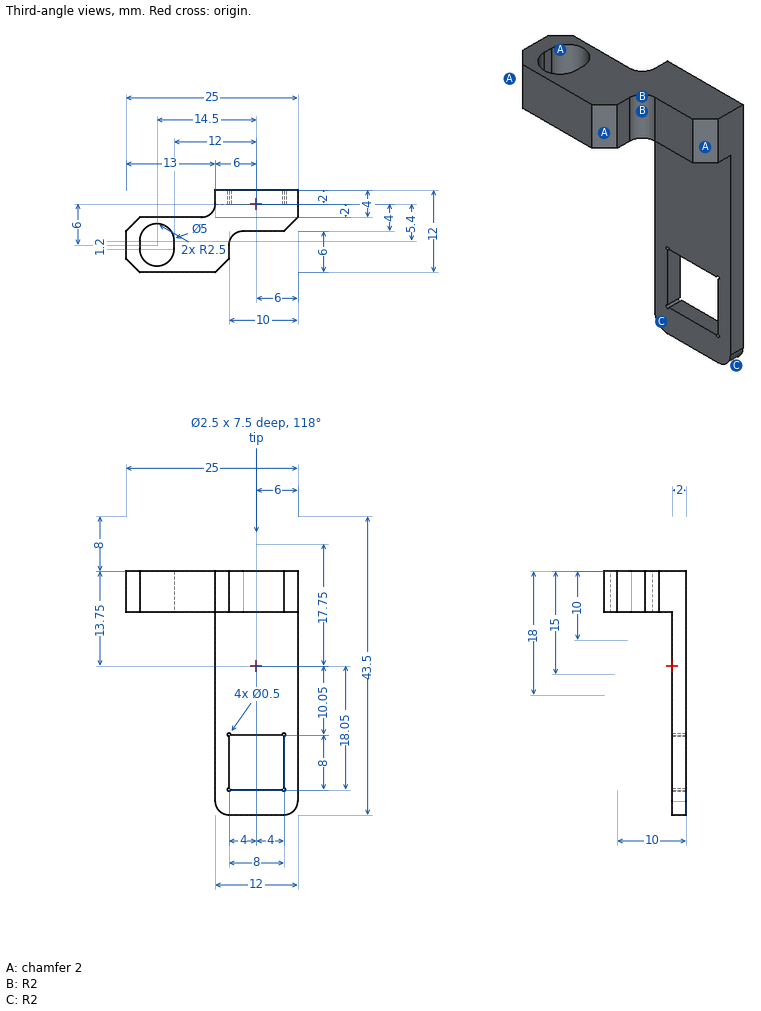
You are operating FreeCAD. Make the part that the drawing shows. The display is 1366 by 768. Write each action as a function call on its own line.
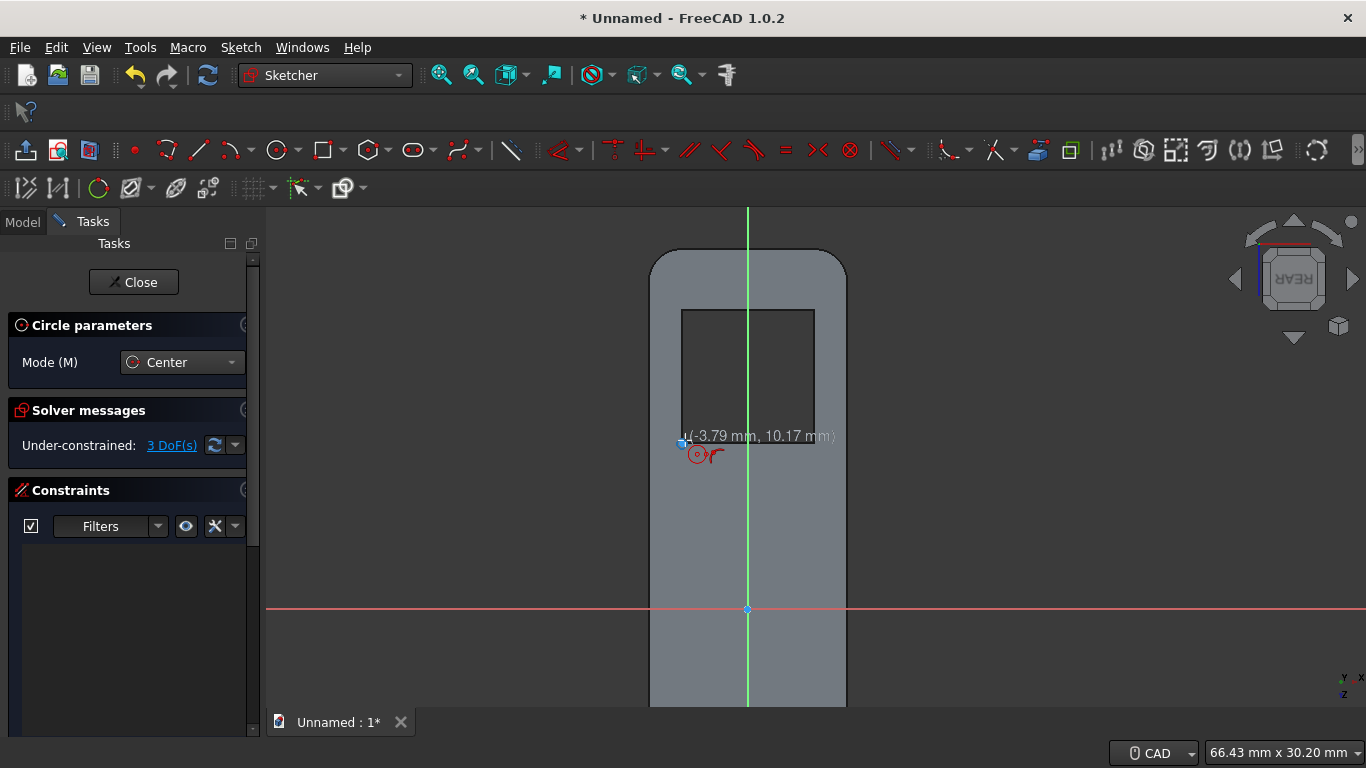
scroll(814, 443, up, 9)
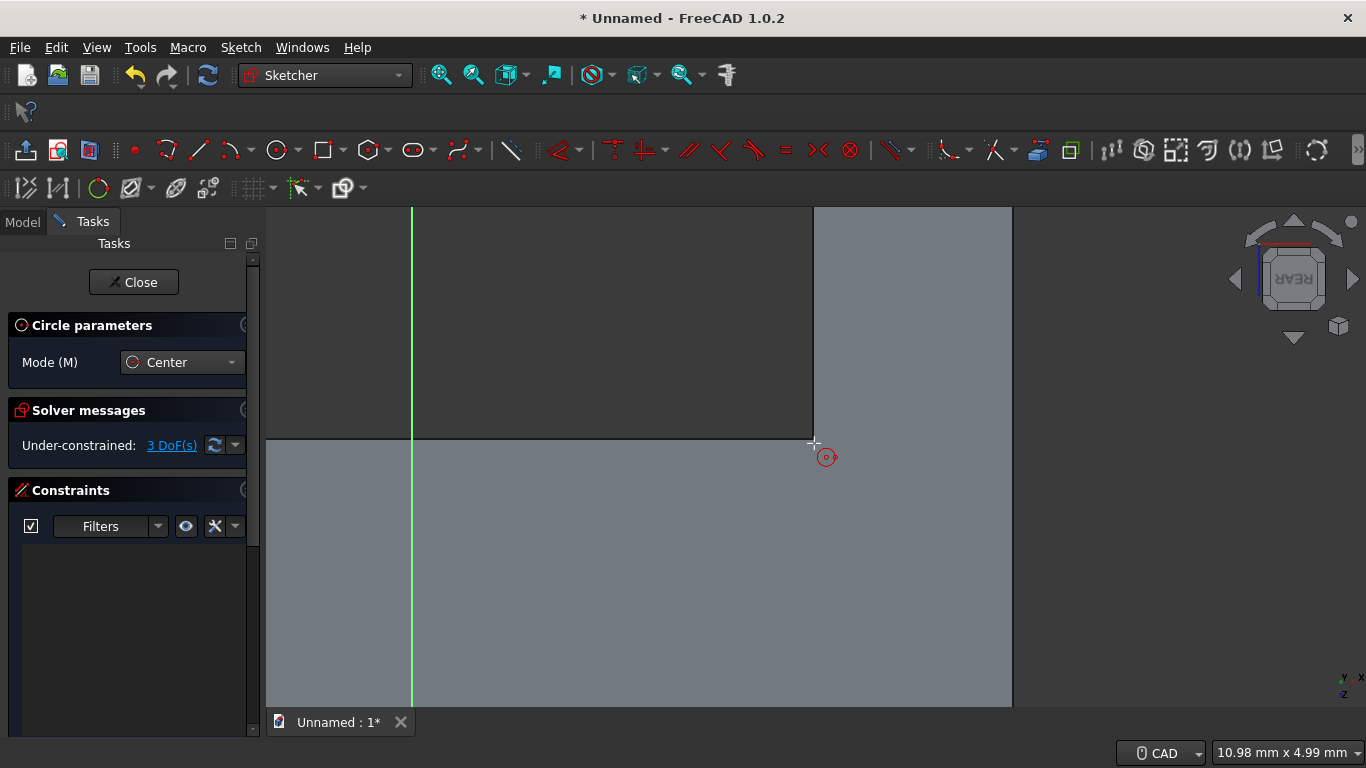
scroll(814, 443, down, 9)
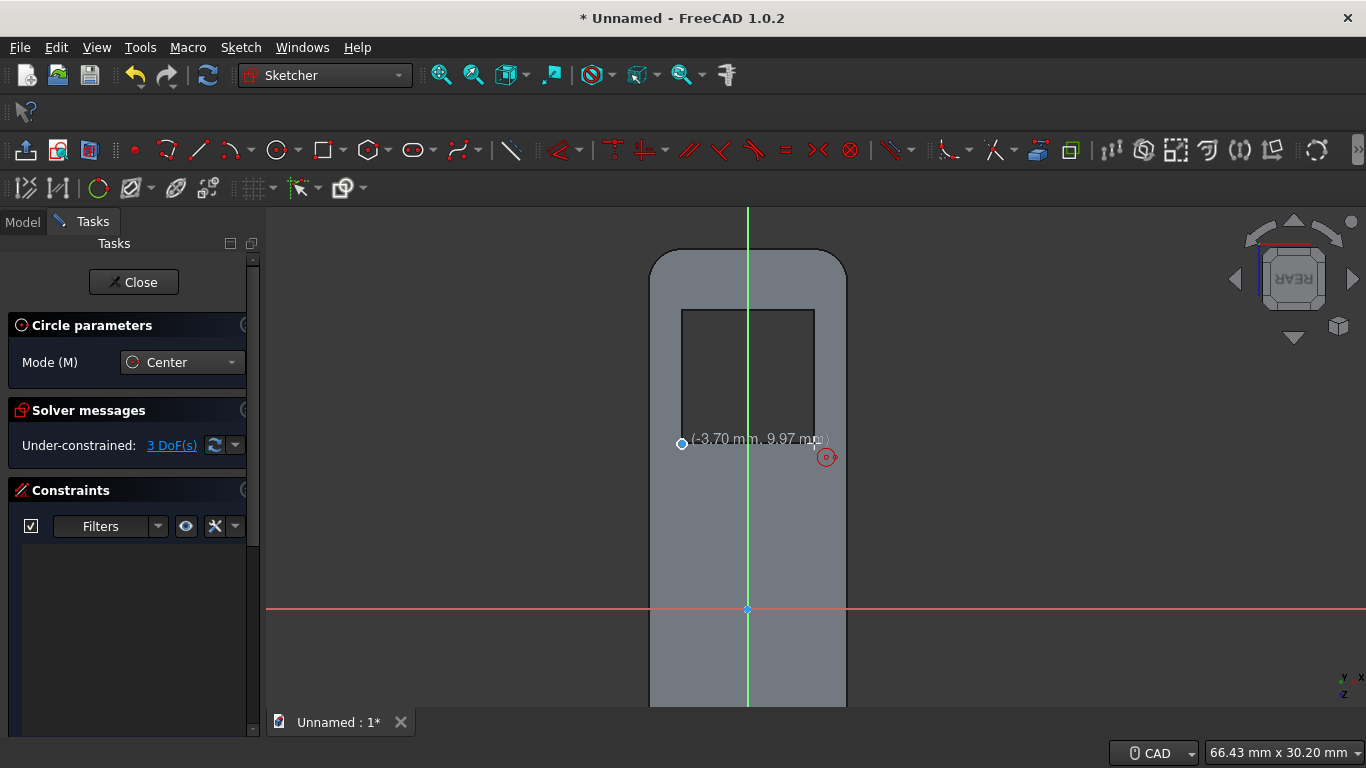
click(814, 443)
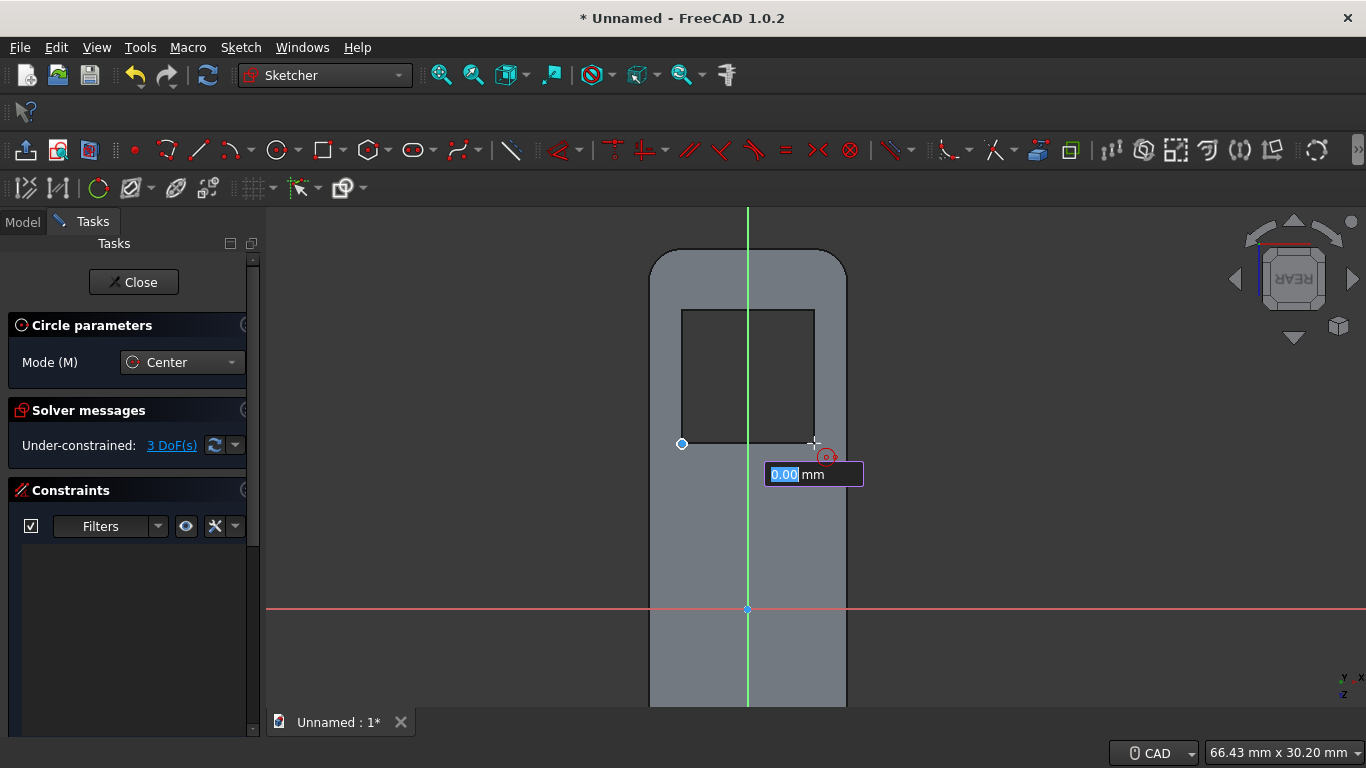
scroll(817, 440, up, 7)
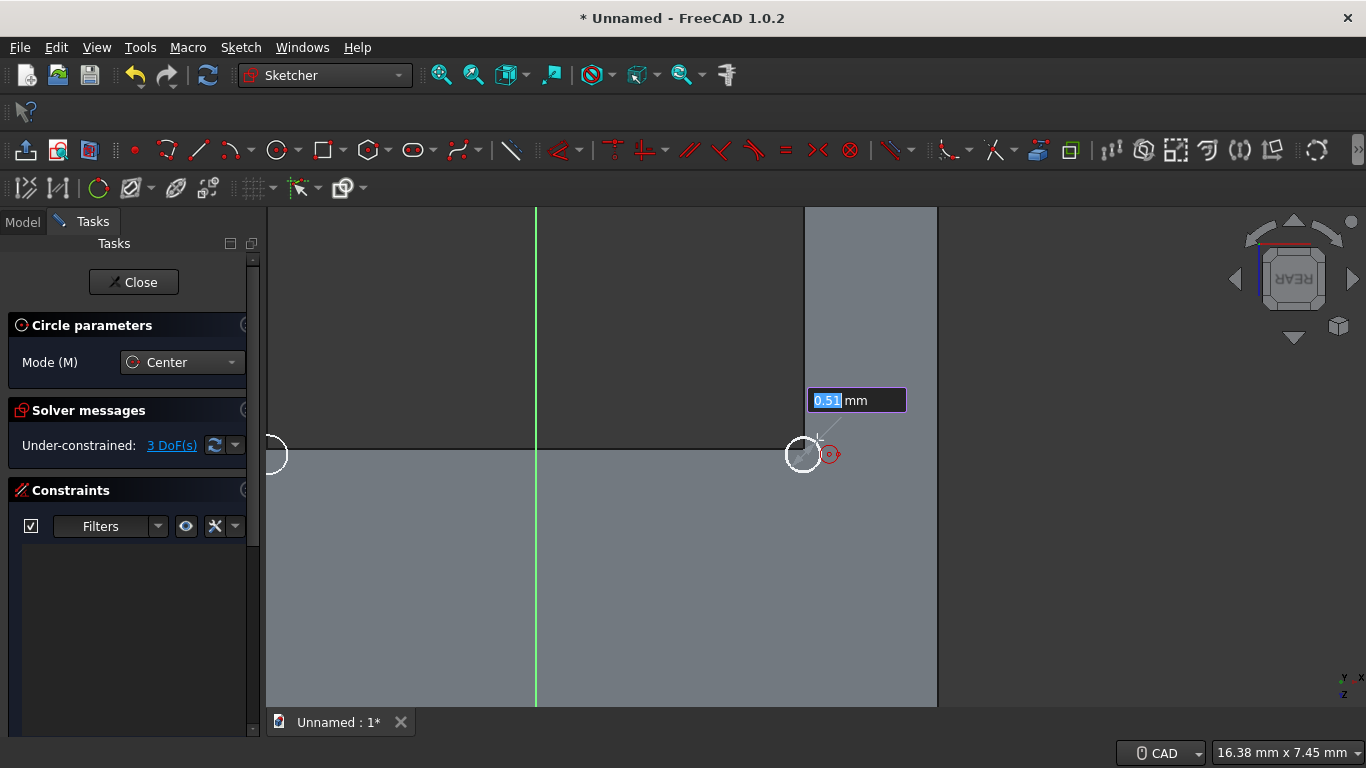
click(816, 438)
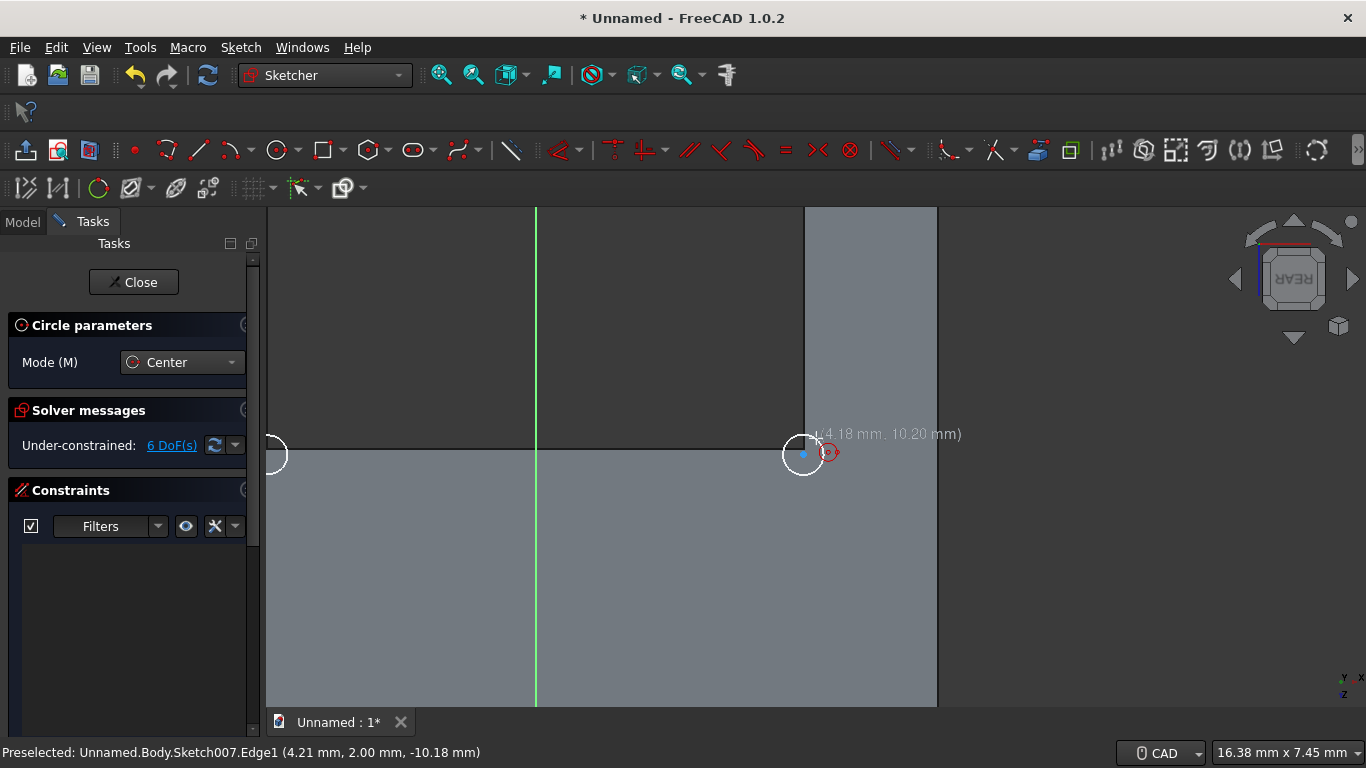
scroll(817, 440, down, 7)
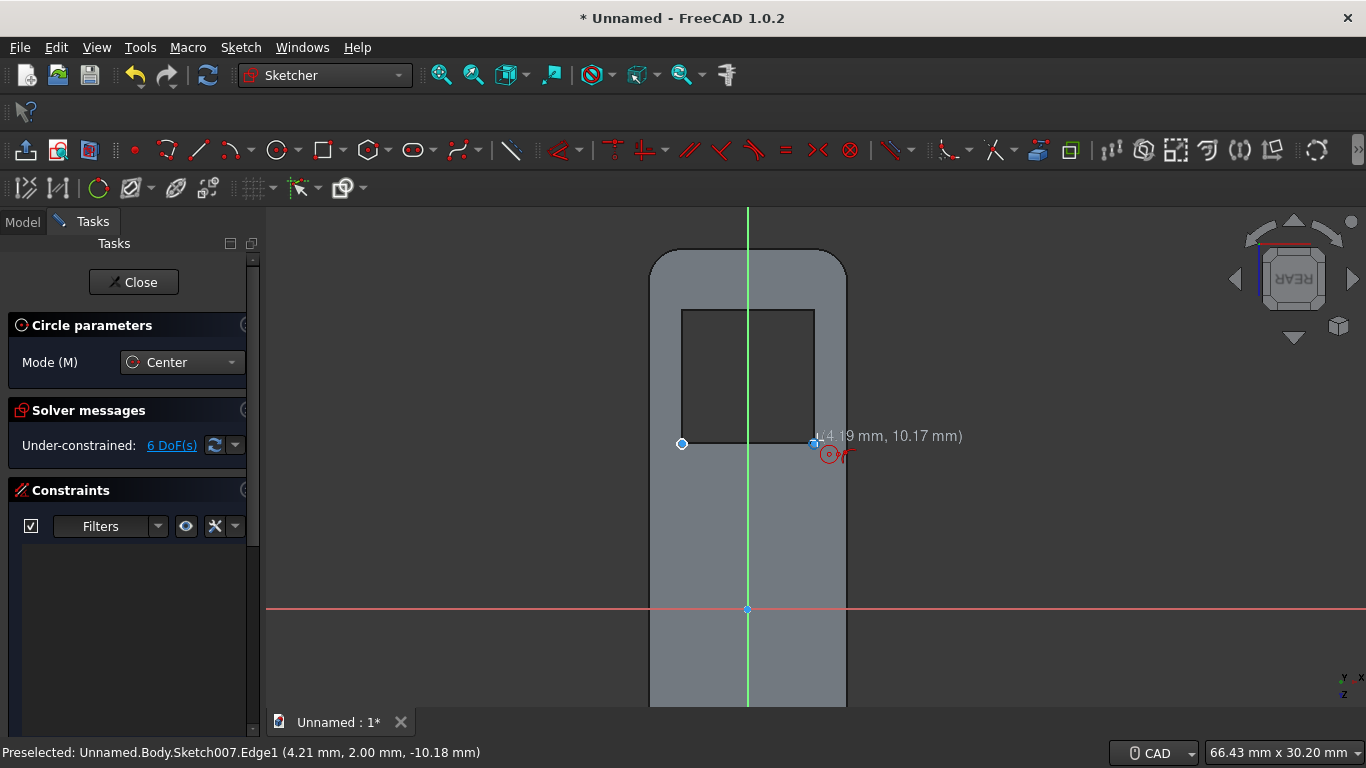
scroll(682, 310, up, 9)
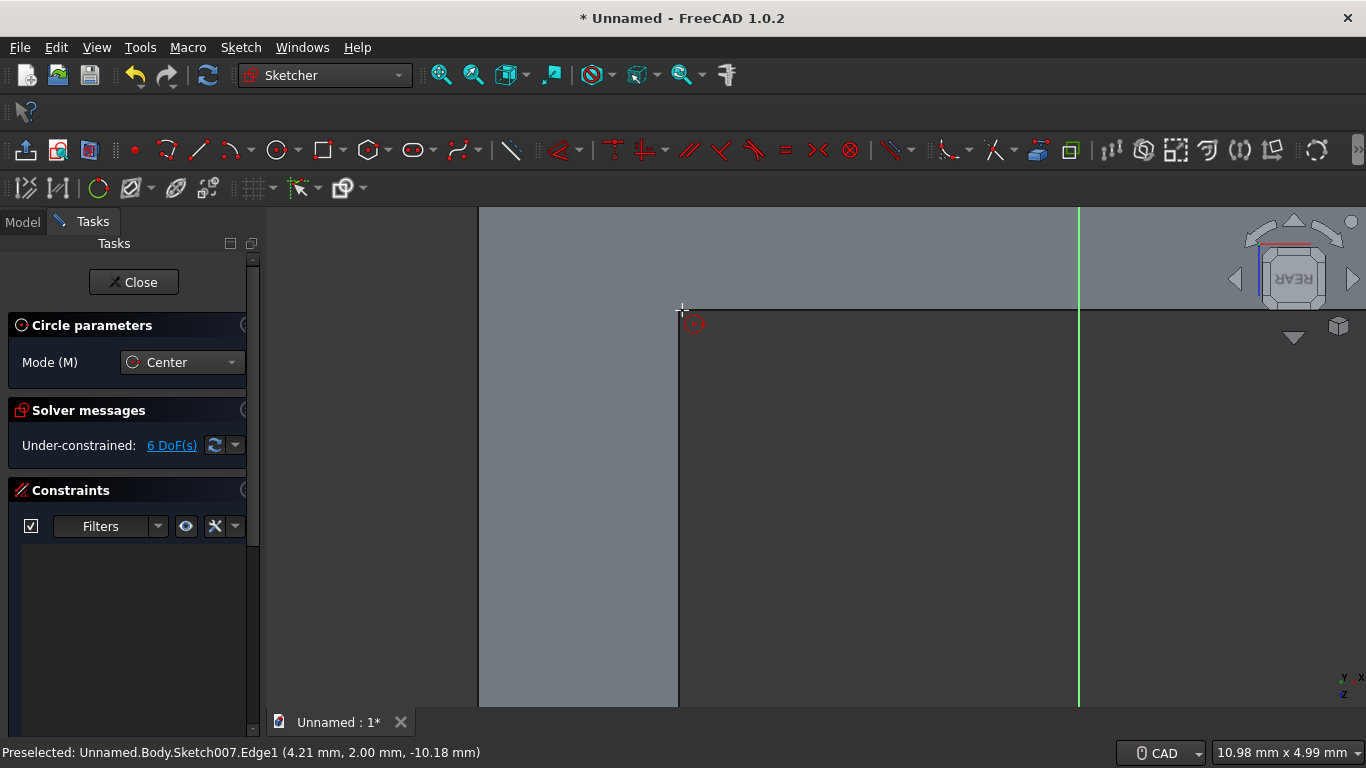
scroll(682, 310, down, 9)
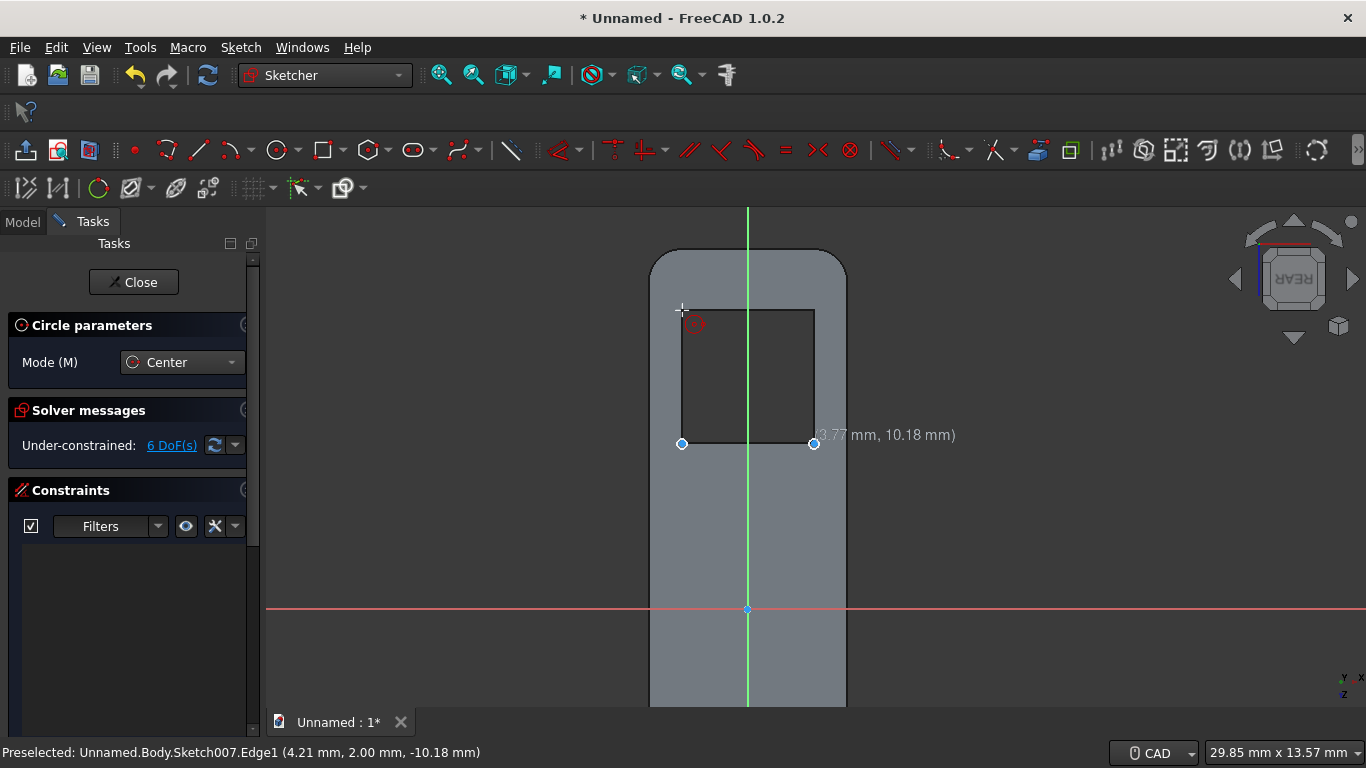
click(682, 310)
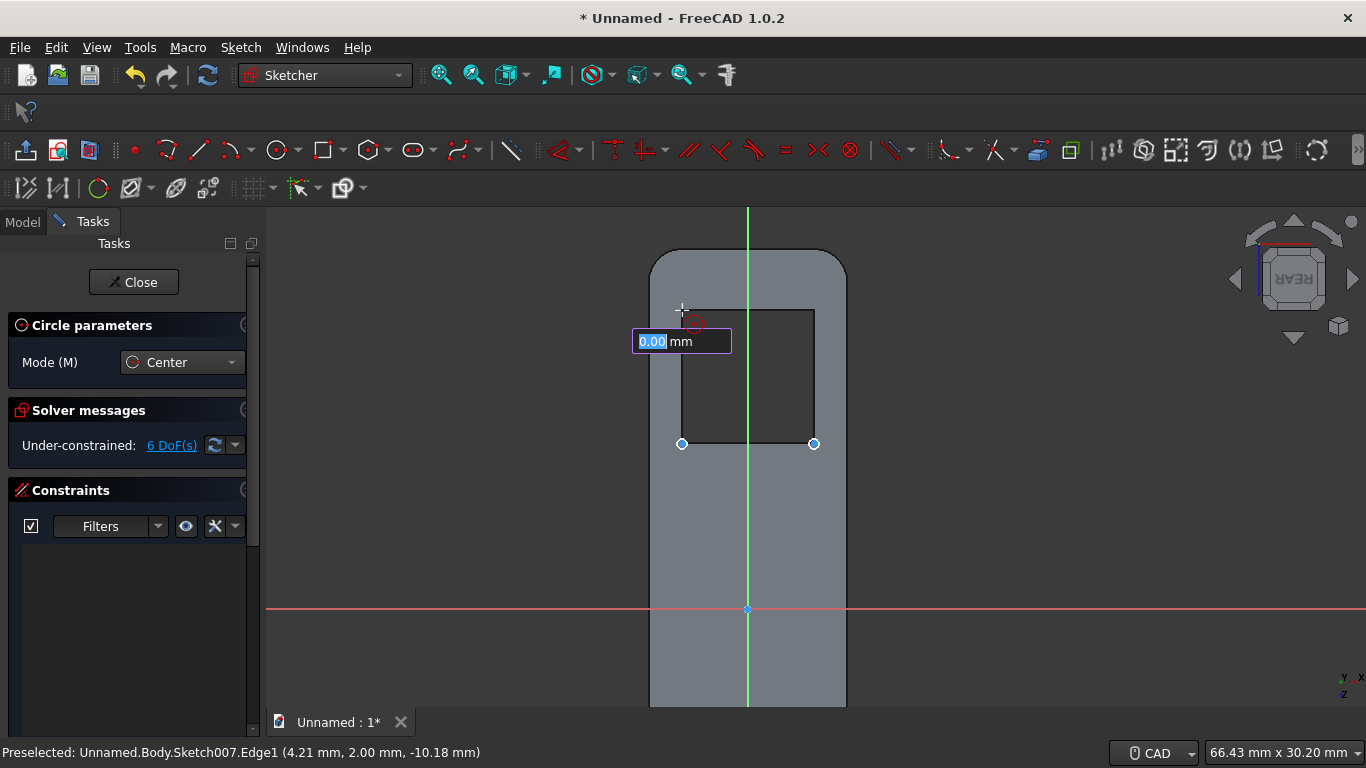
scroll(685, 307, up, 7)